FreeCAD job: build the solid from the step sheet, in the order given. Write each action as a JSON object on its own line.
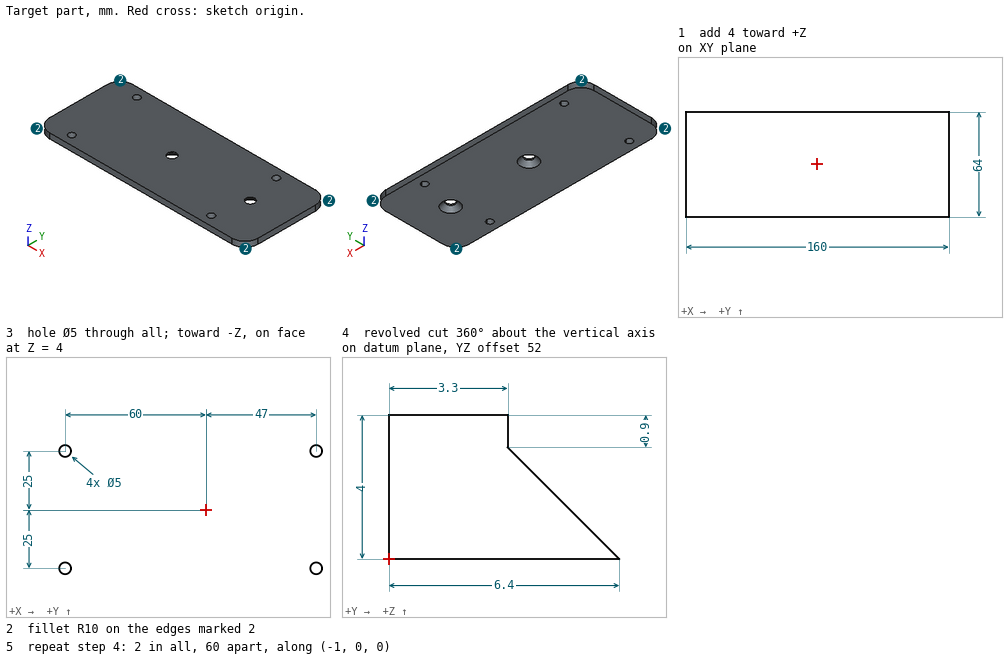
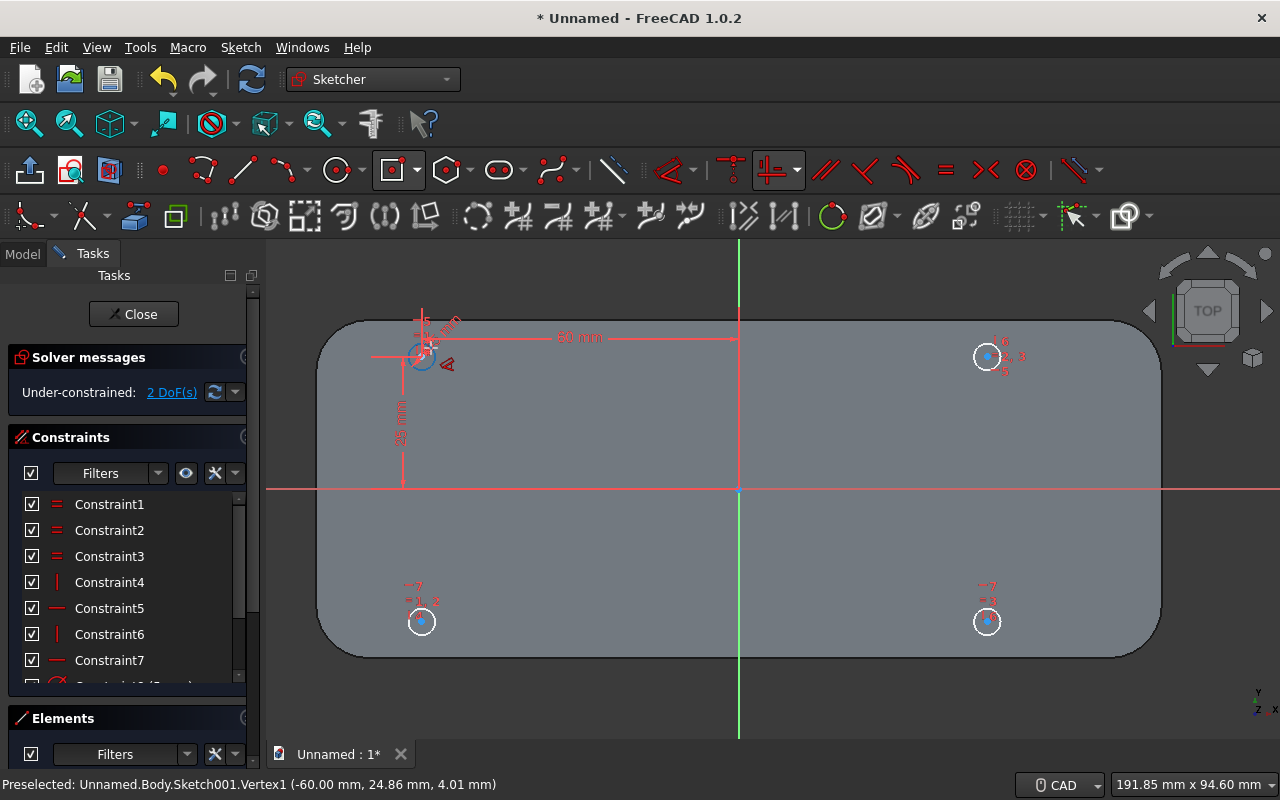
{"action": "left_click", "coordinate": [422, 622]}
{"action": "left_click", "coordinate": [388, 555]}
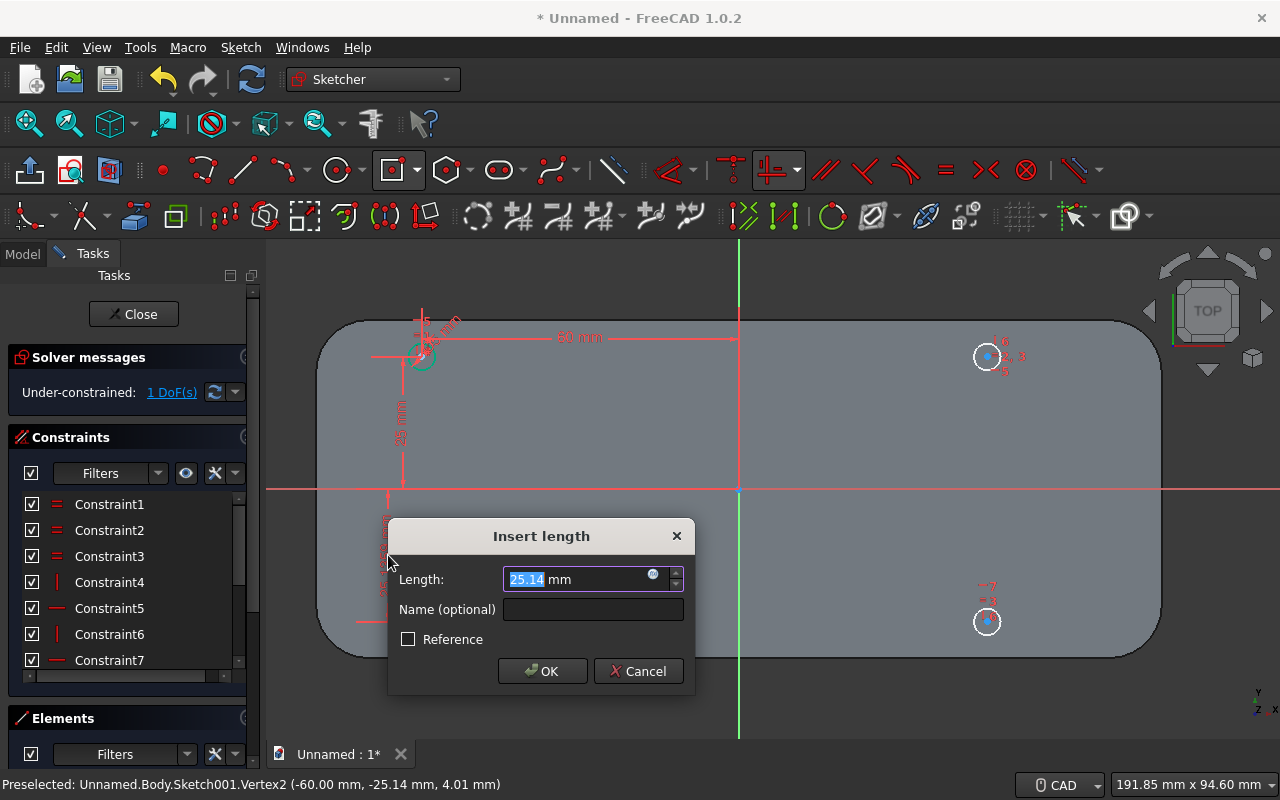
{"action": "type", "text": "25"}
{"action": "key", "text": "Return"}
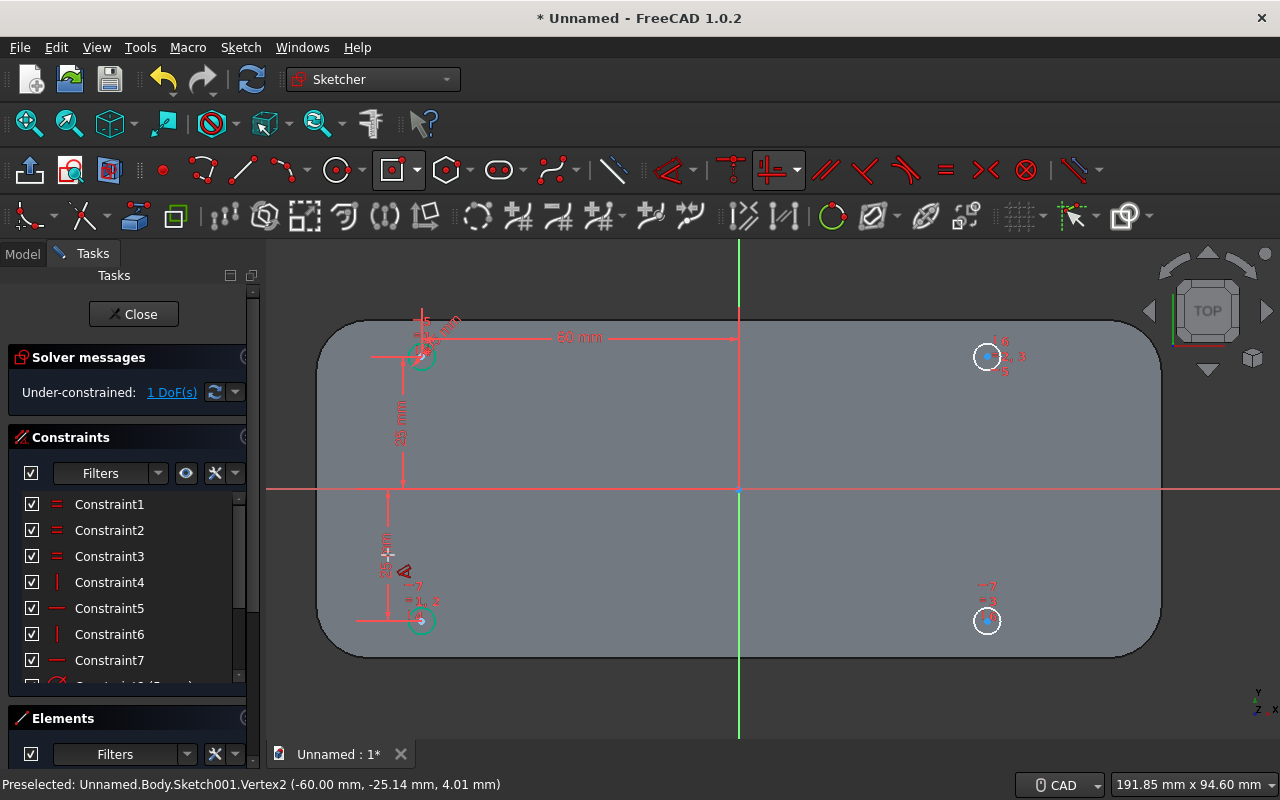
{"action": "left_click", "coordinate": [987, 357]}
{"action": "left_click", "coordinate": [863, 323]}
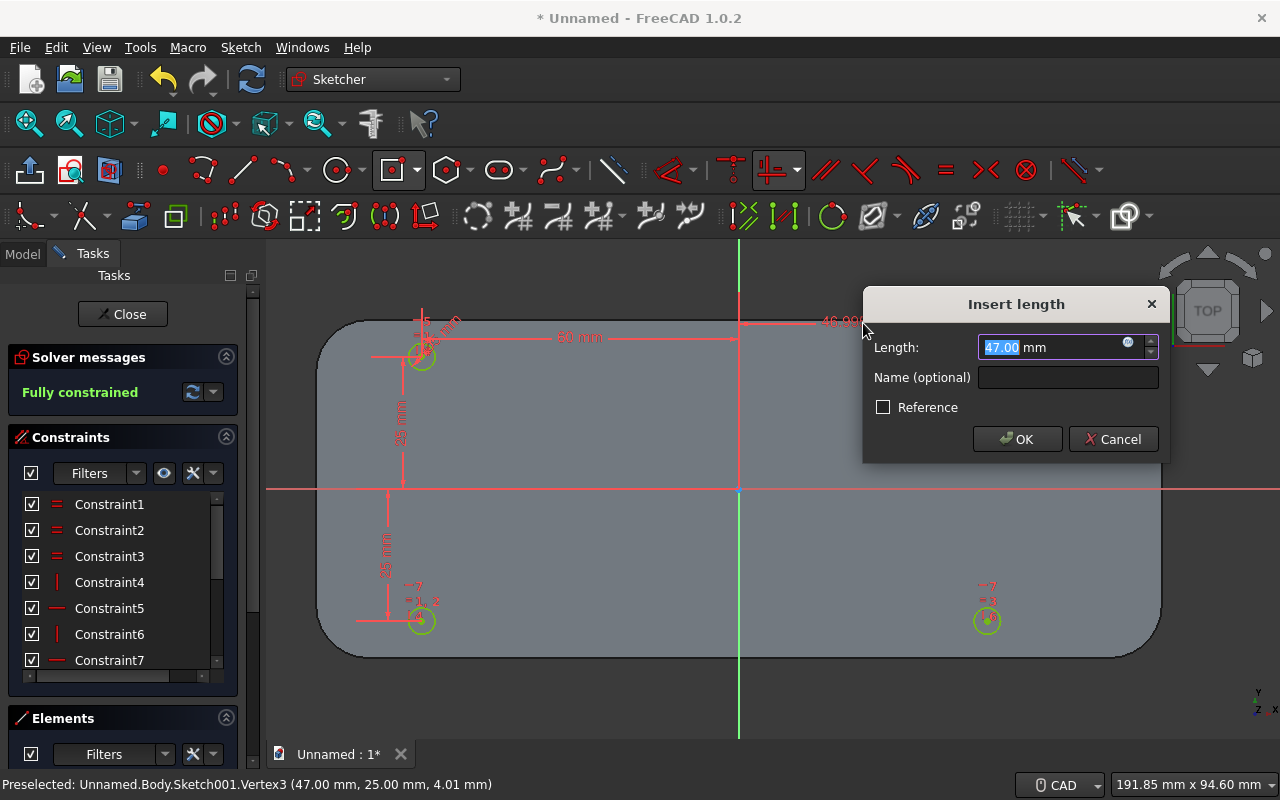
{"action": "type", "text": "47"}
{"action": "key", "text": "Return"}
{"action": "key", "text": "Escape"}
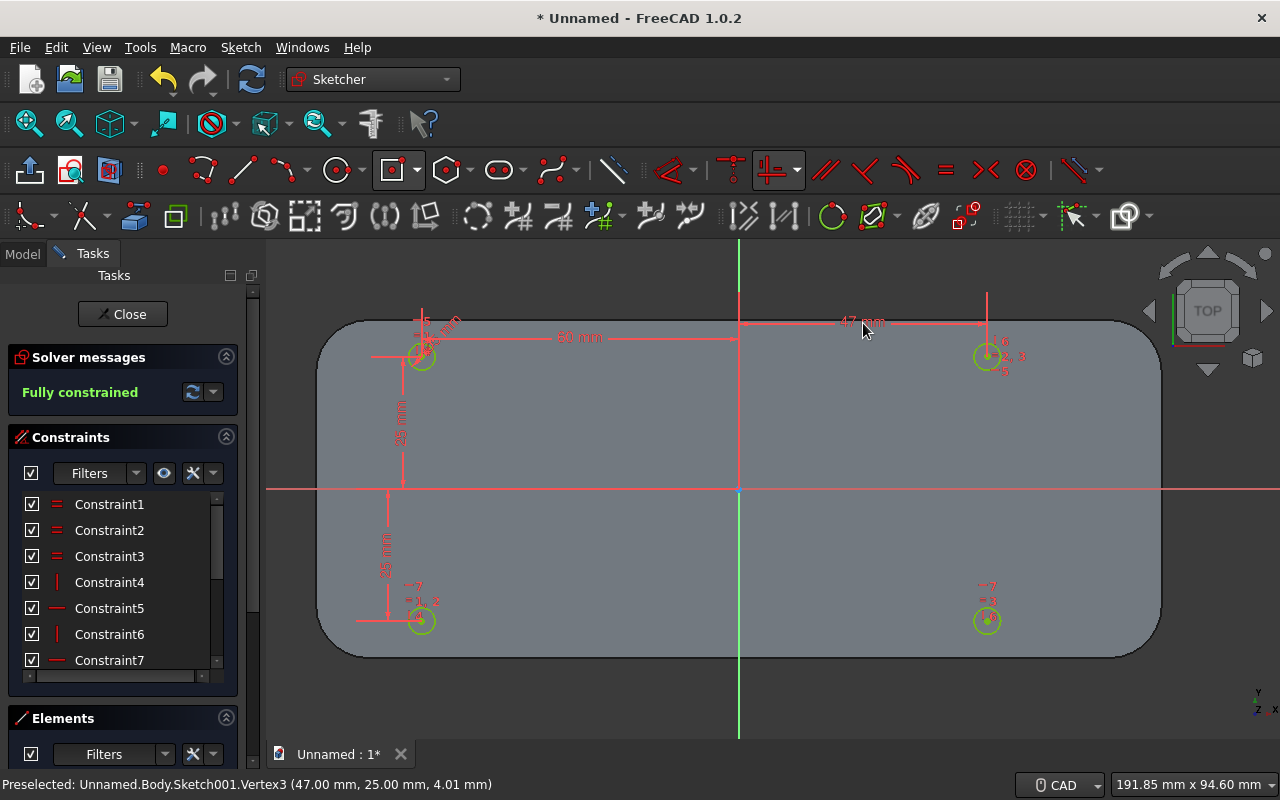
{"action": "left_click", "coordinate": [123, 314]}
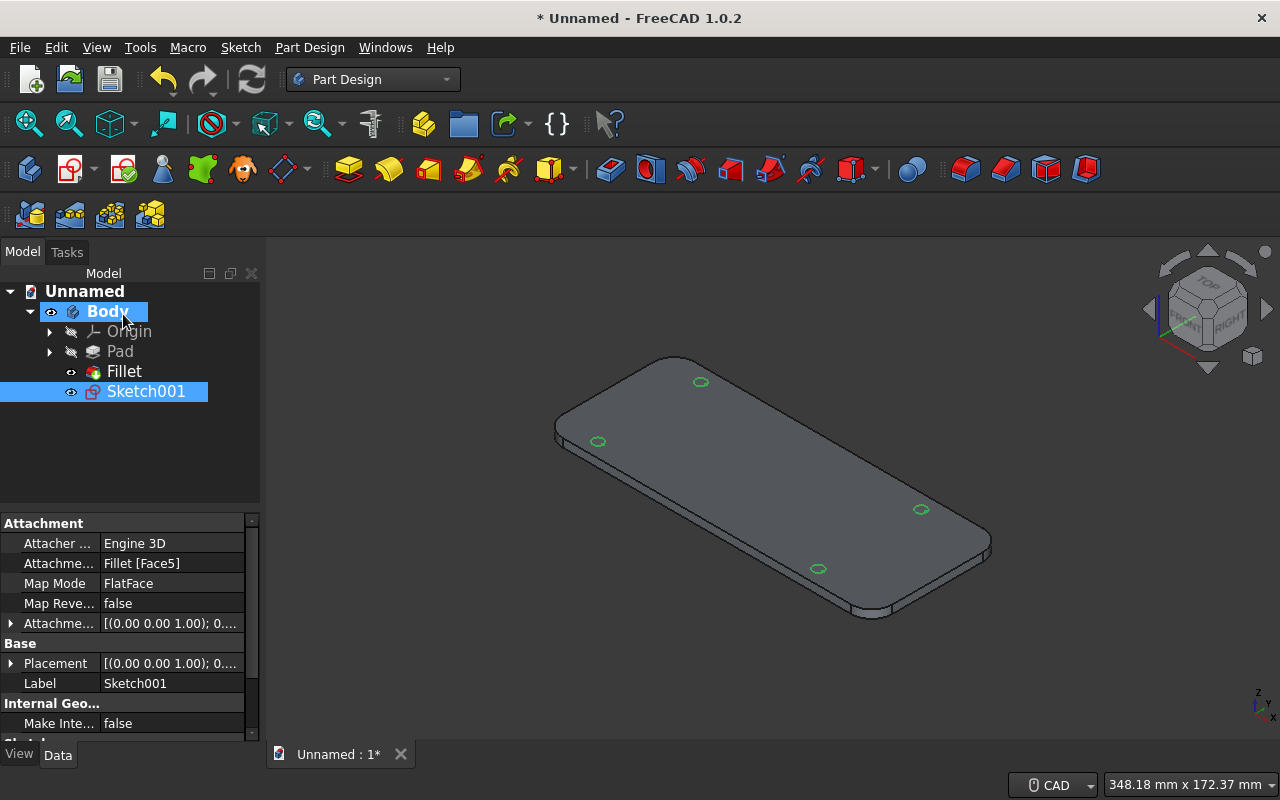
{"action": "left_click", "coordinate": [652, 170]}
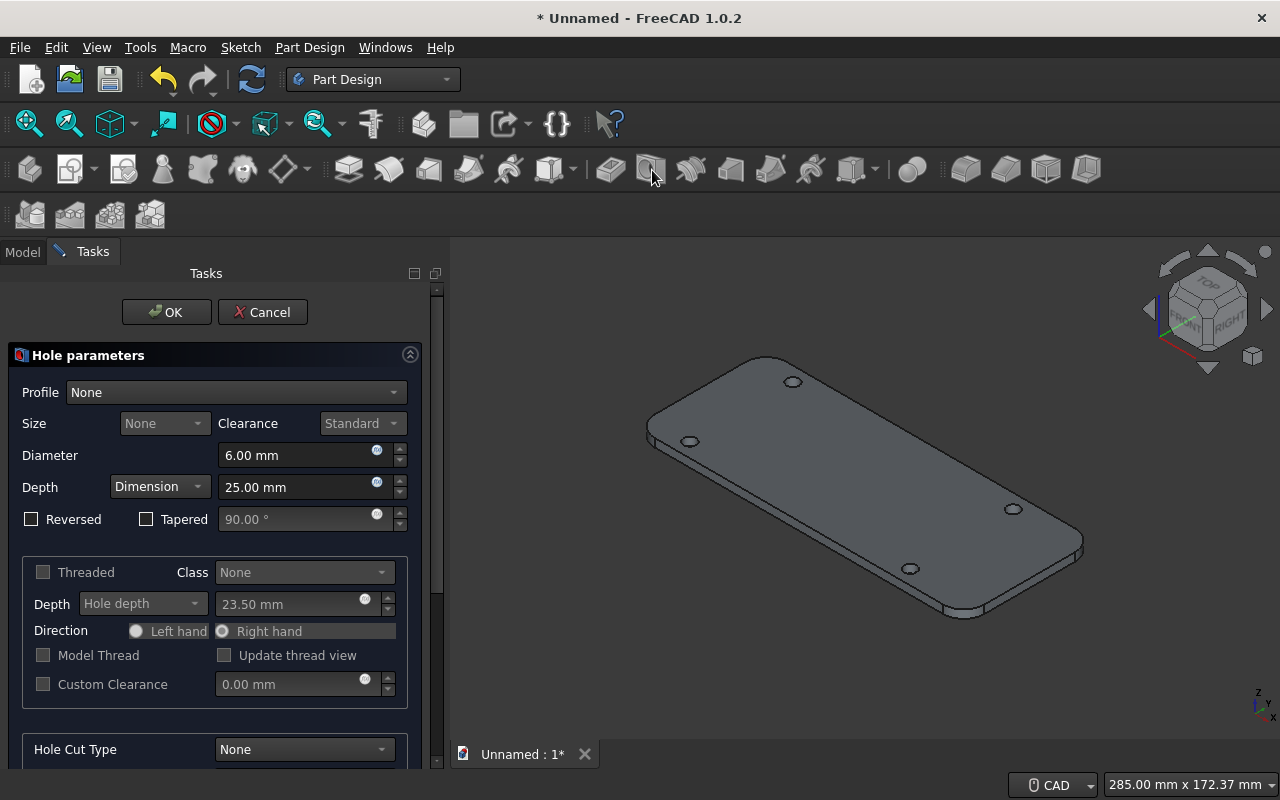
{"action": "triple_click", "coordinate": [305, 455]}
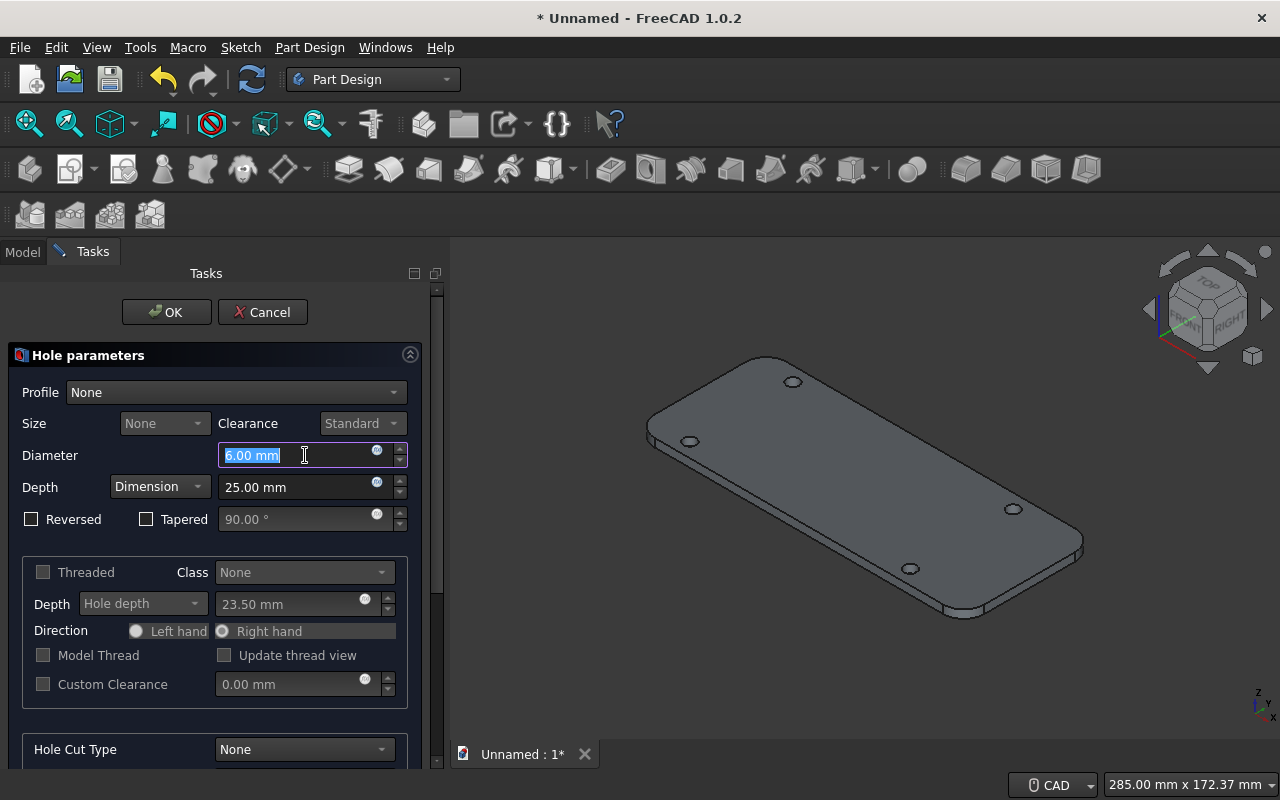
{"action": "type", "text": "5"}
{"action": "key", "text": "Tab"}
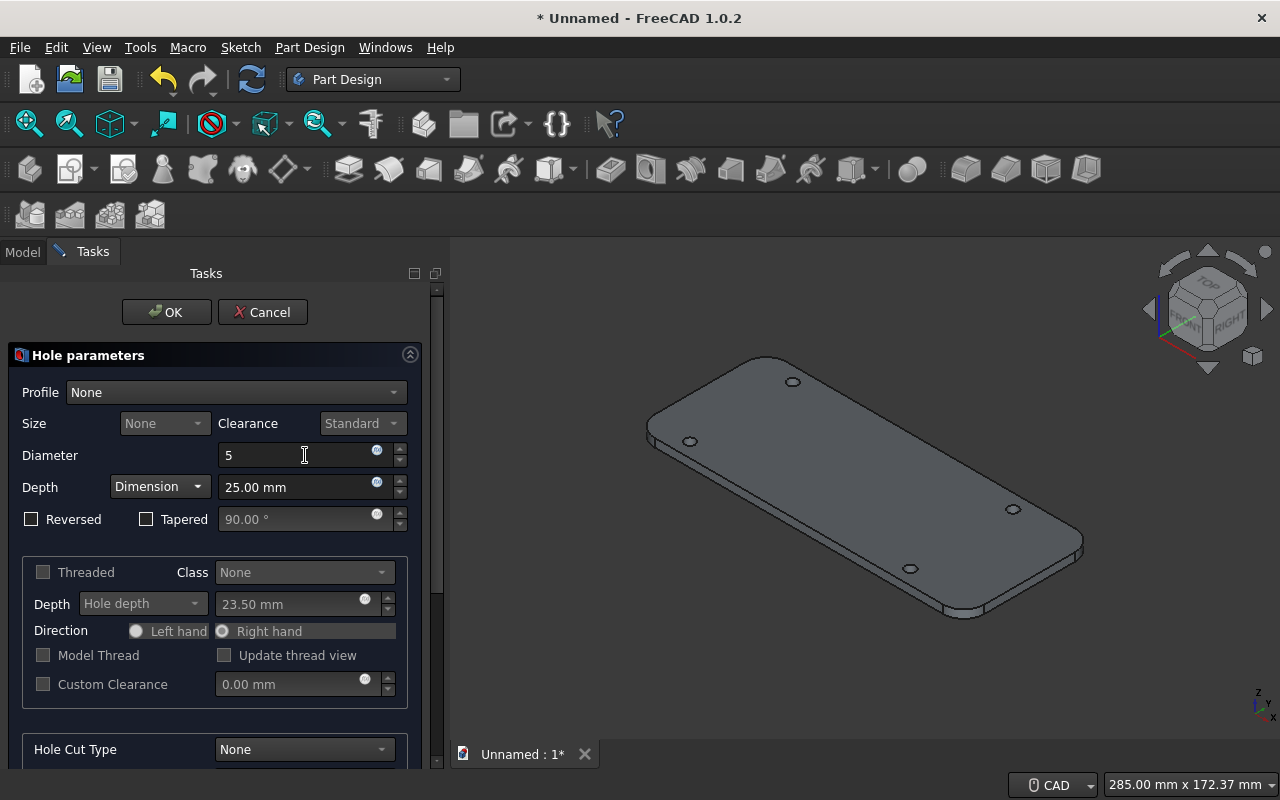
{"action": "left_click", "coordinate": [161, 486]}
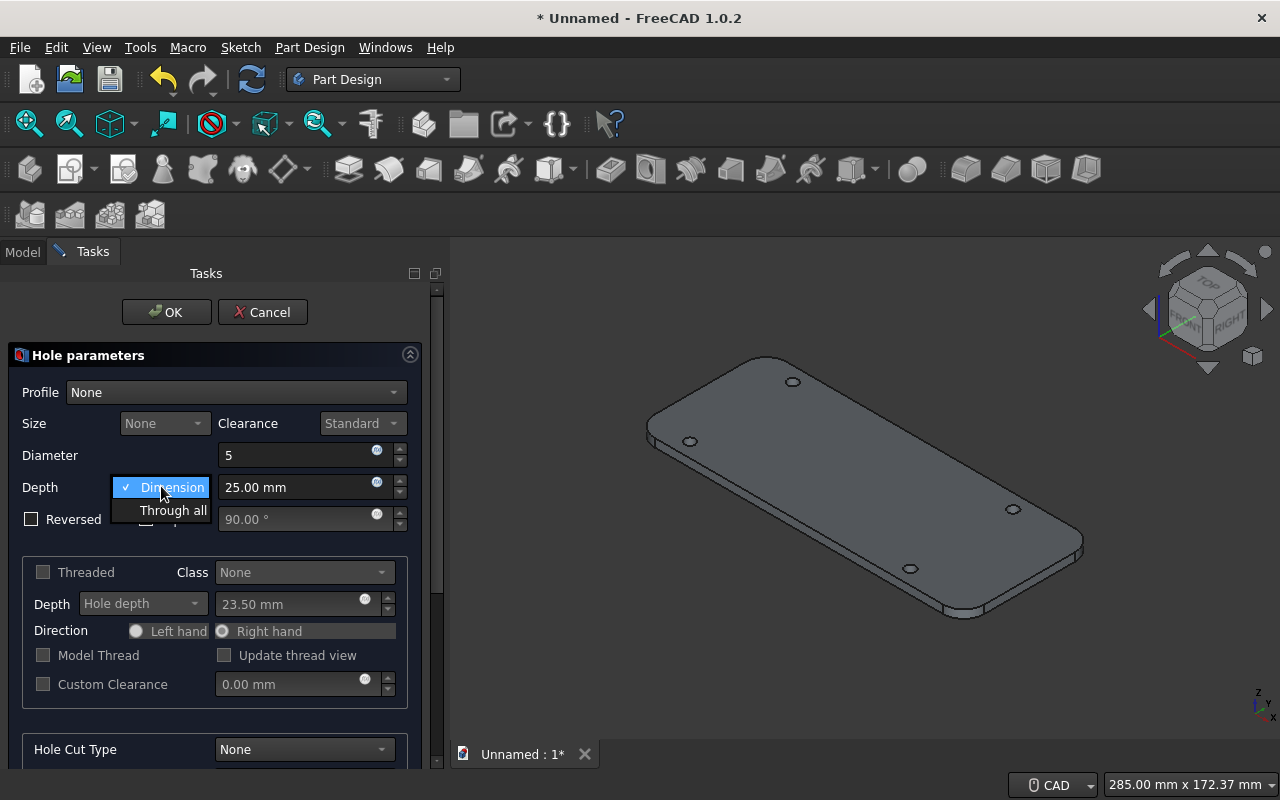
{"action": "left_click", "coordinate": [160, 510]}